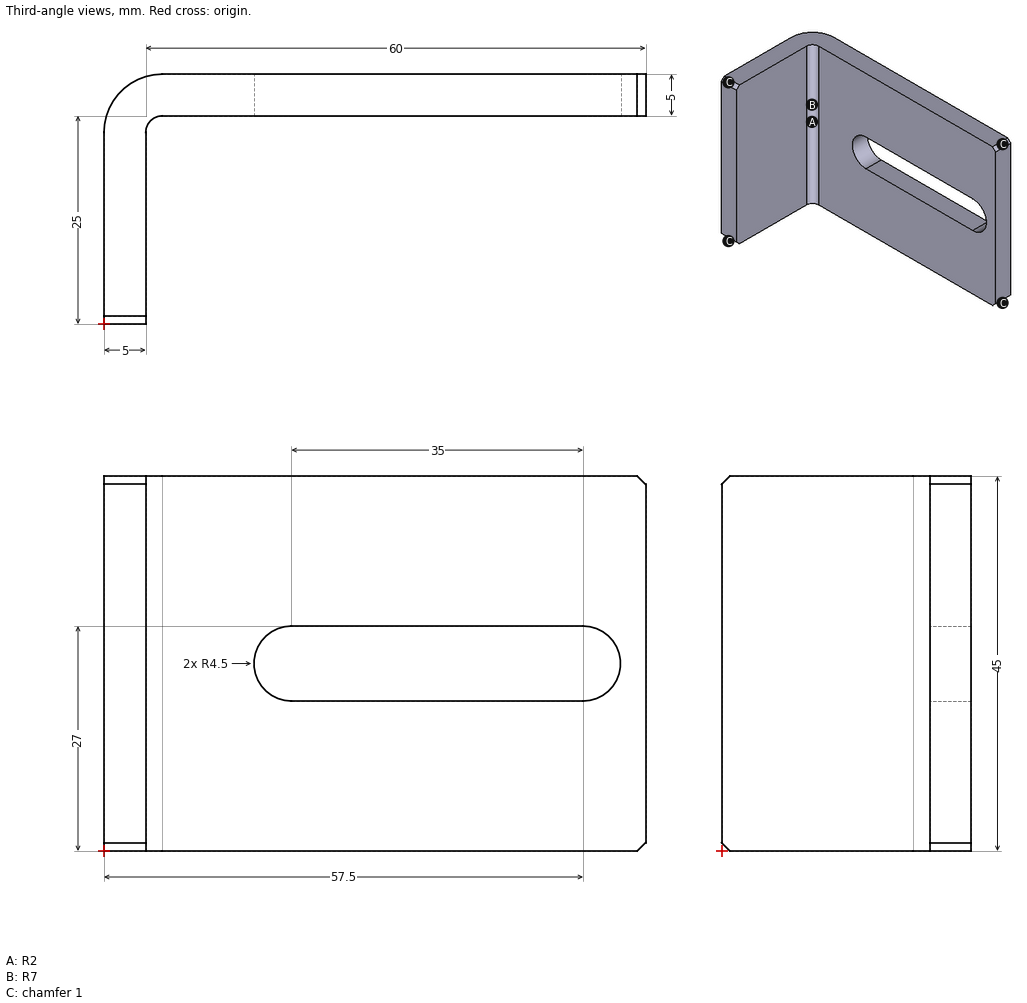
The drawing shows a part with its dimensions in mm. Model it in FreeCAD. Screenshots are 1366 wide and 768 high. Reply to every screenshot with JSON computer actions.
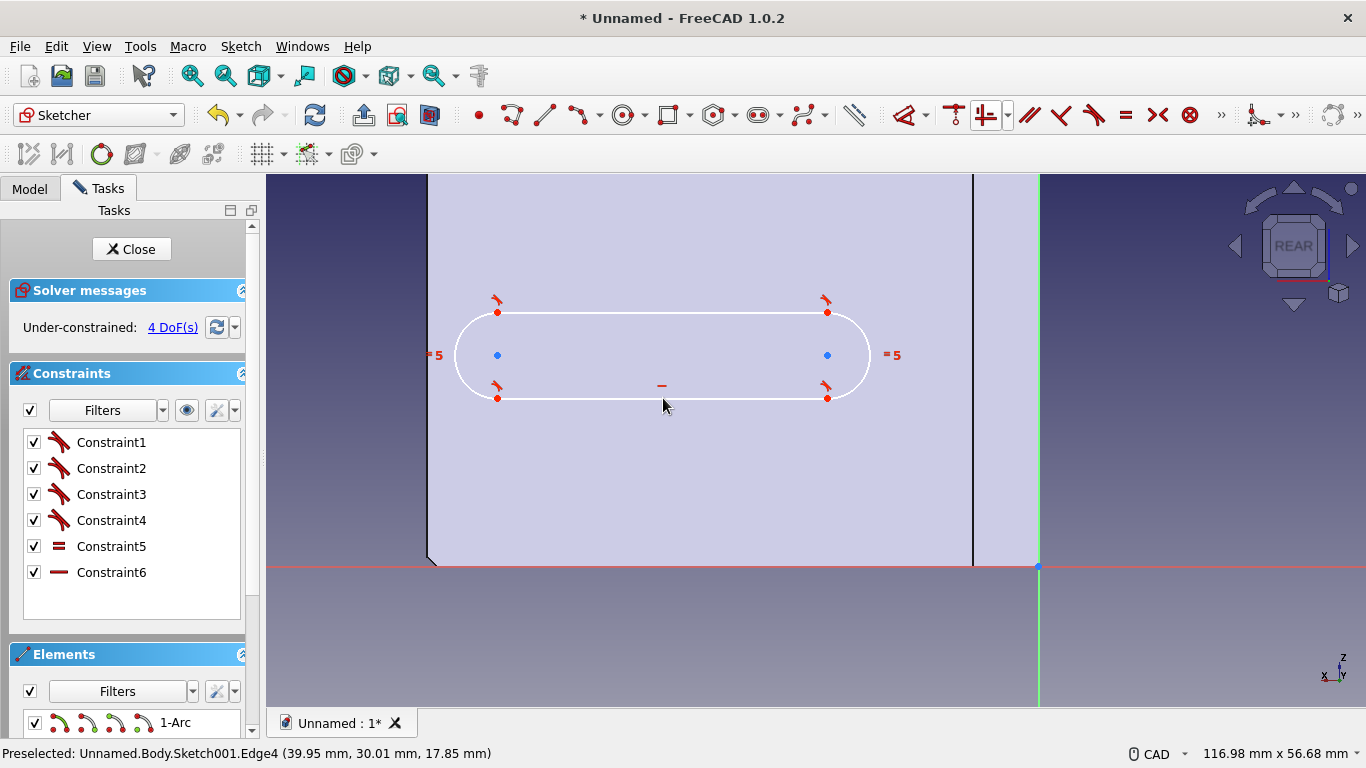
{"action": "key", "text": "d"}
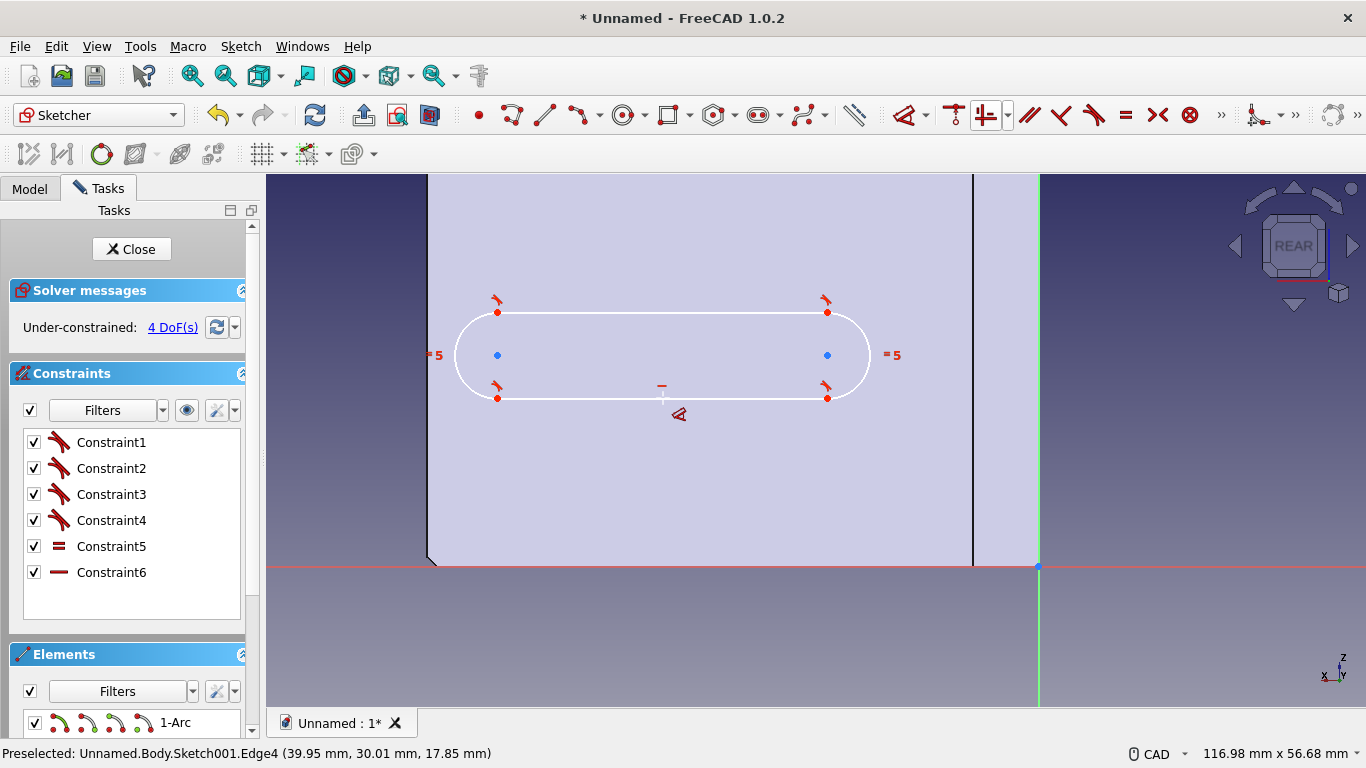
{"action": "left_click", "coordinate": [463, 331]}
{"action": "left_click", "coordinate": [437, 312]}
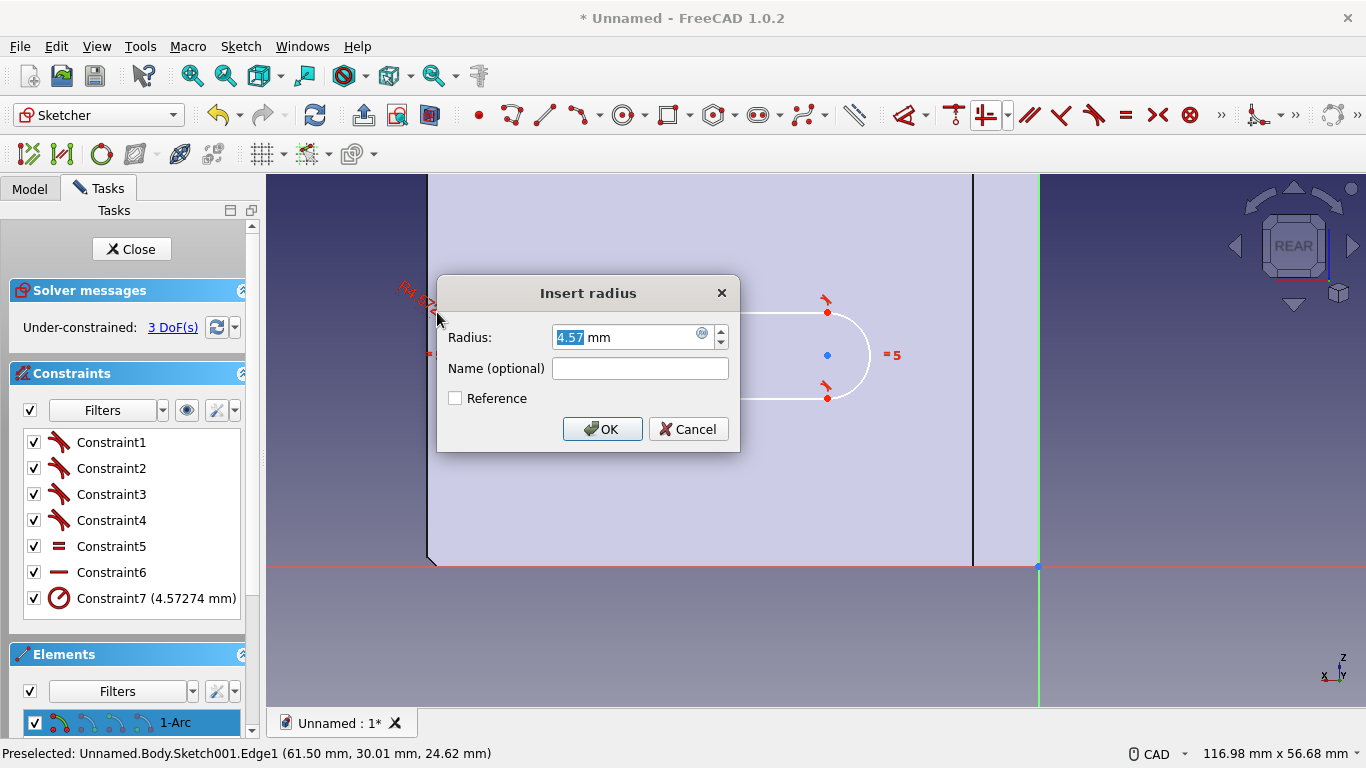
{"action": "type", "text": "4.5"}
{"action": "key", "text": "Return"}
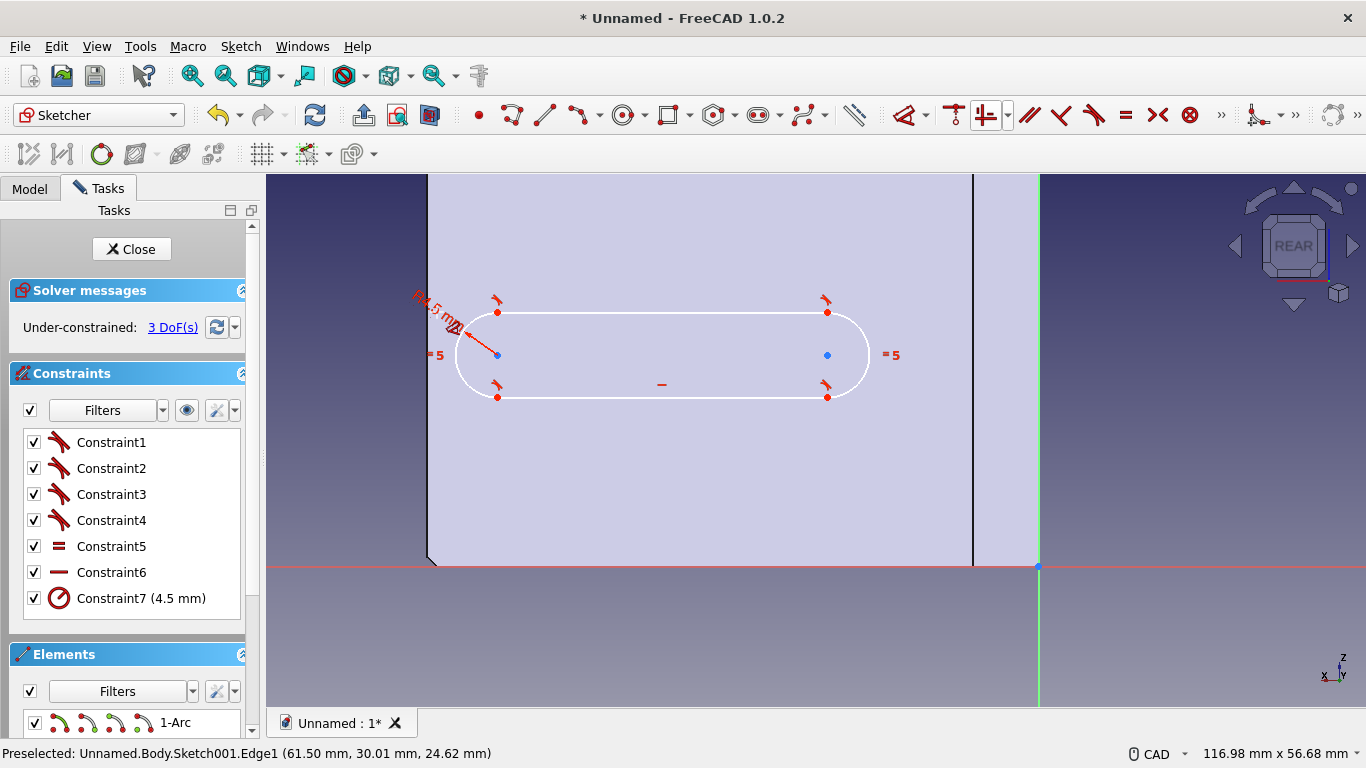
{"action": "left_click", "coordinate": [597, 313]}
{"action": "left_click", "coordinate": [662, 279]}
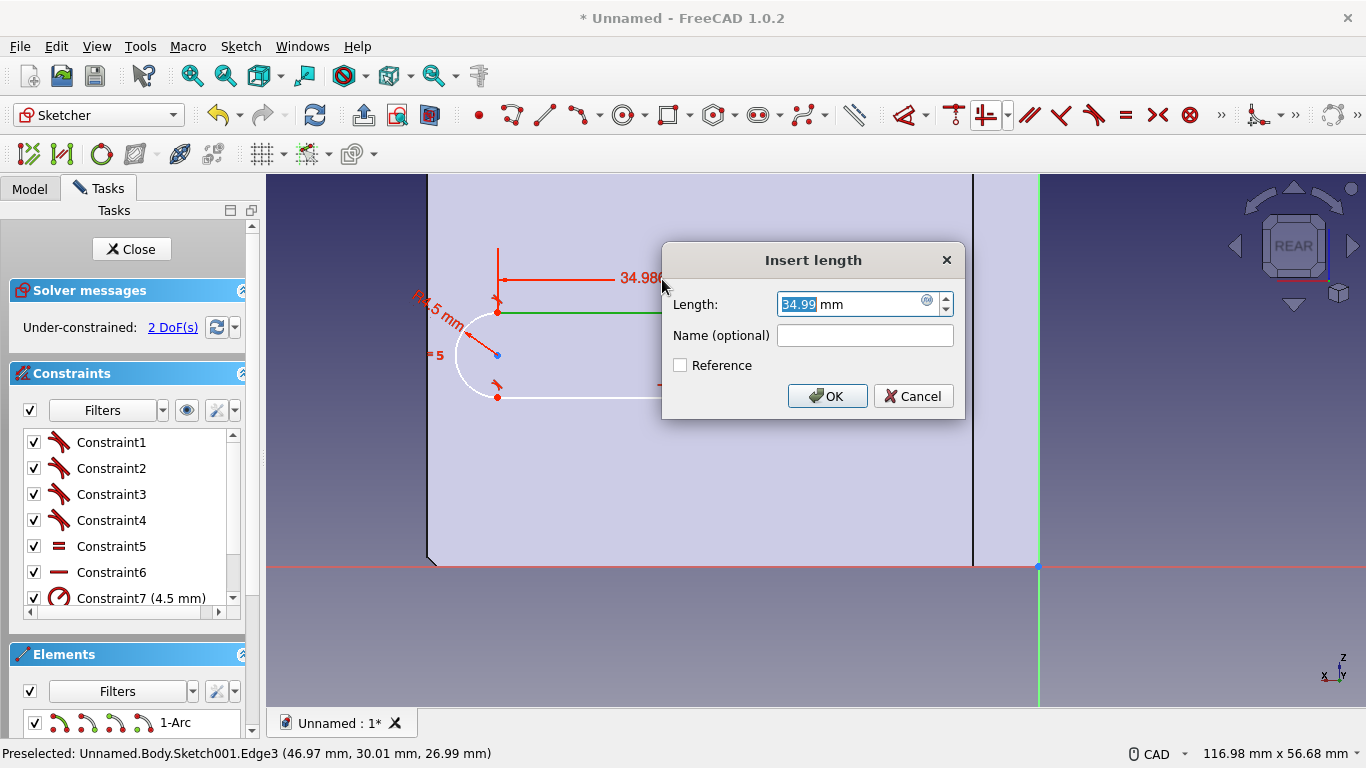
{"action": "type", "text": "35"}
{"action": "key", "text": "Return"}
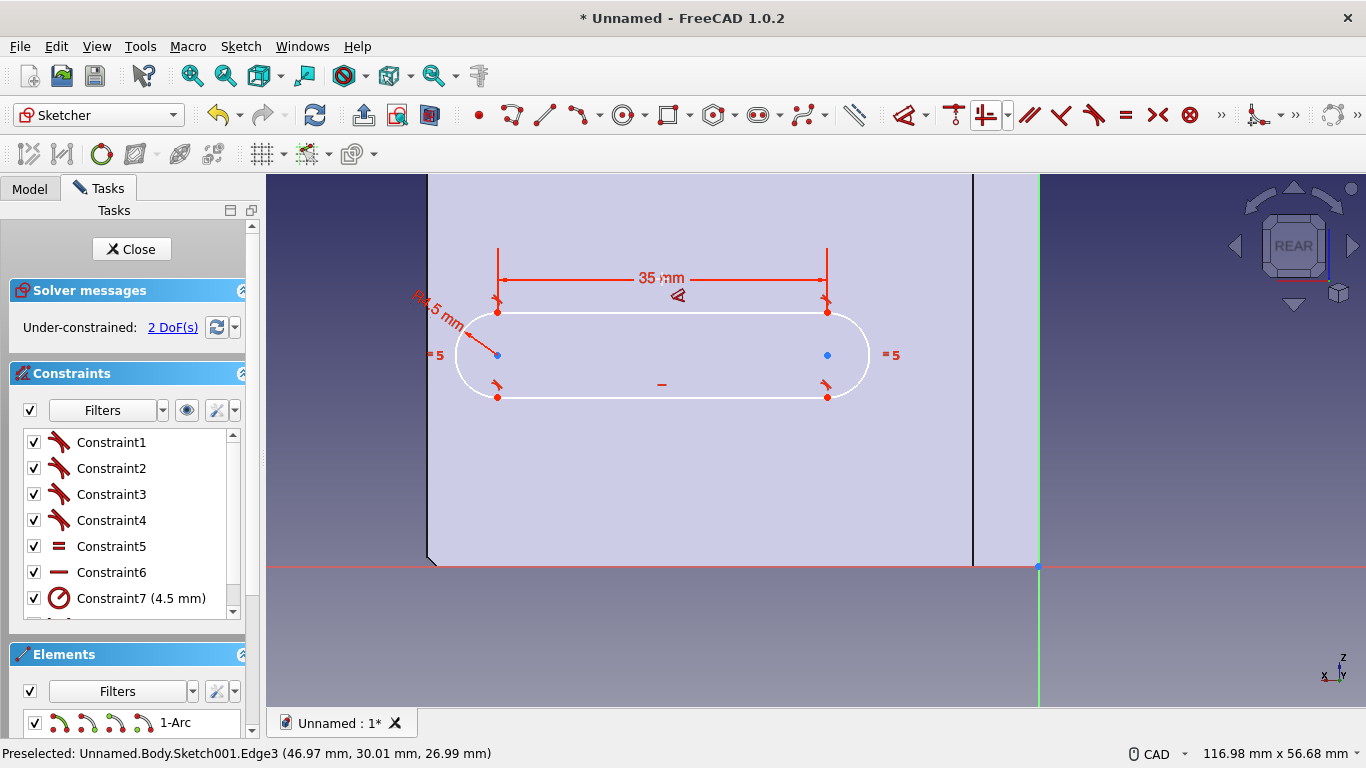
{"action": "left_click", "coordinate": [498, 313]}
{"action": "left_click", "coordinate": [1073, 440]}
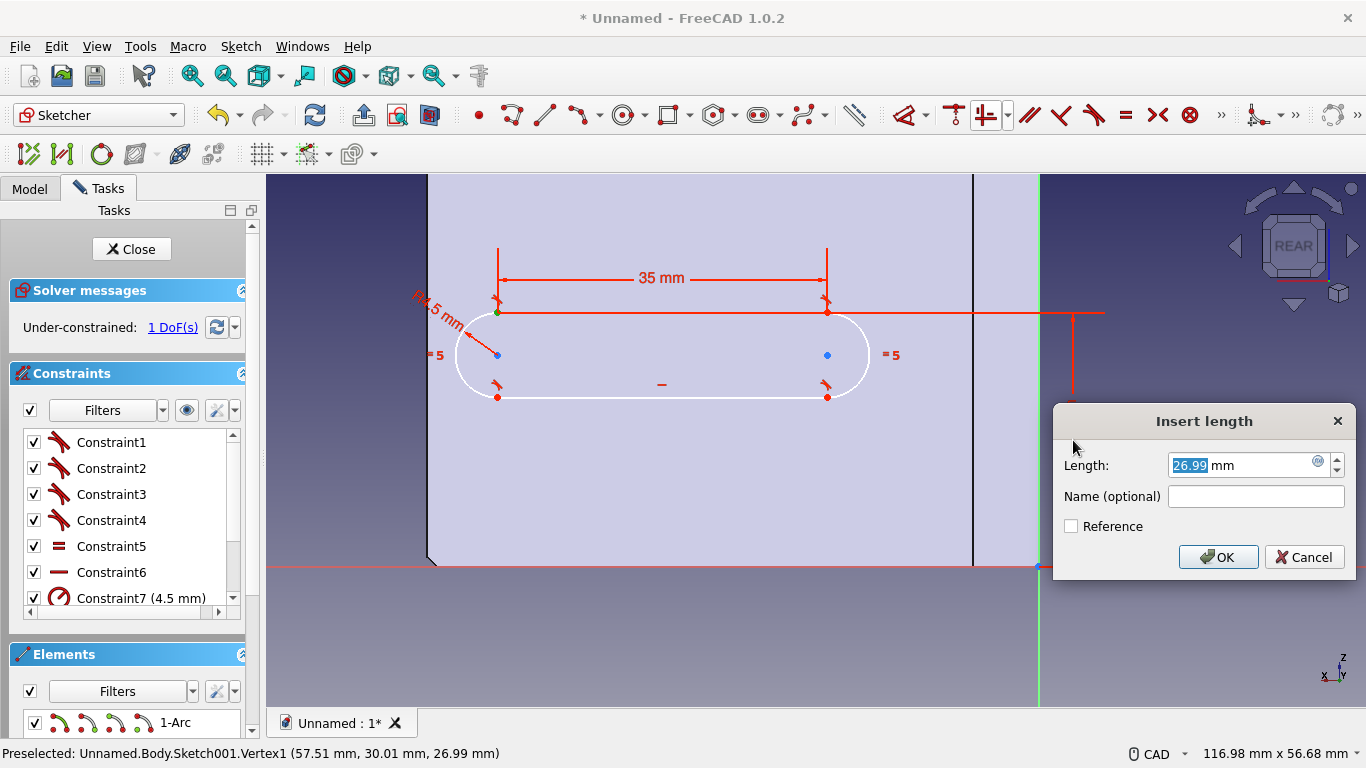
{"action": "type", "text": "27"}
{"action": "key", "text": "Return"}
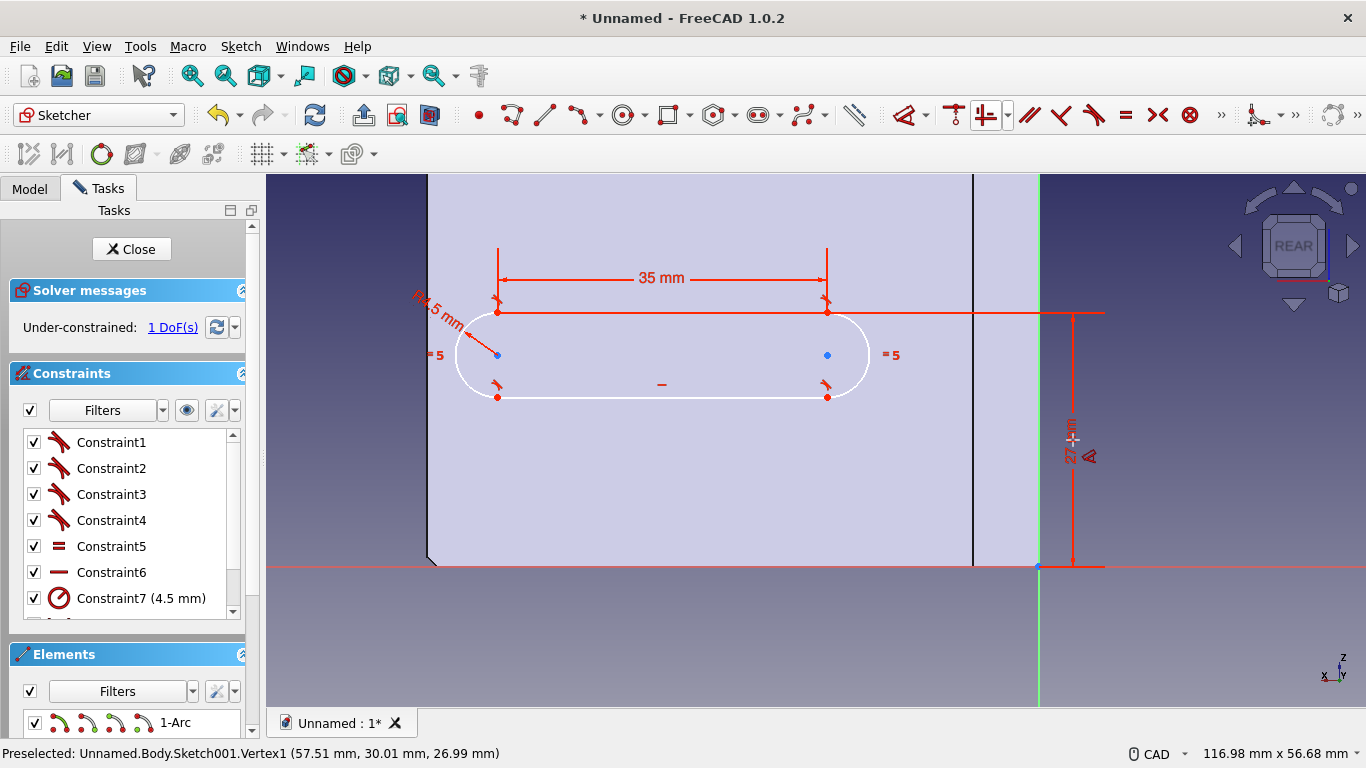
{"action": "left_click", "coordinate": [498, 313]}
{"action": "left_click", "coordinate": [768, 601]}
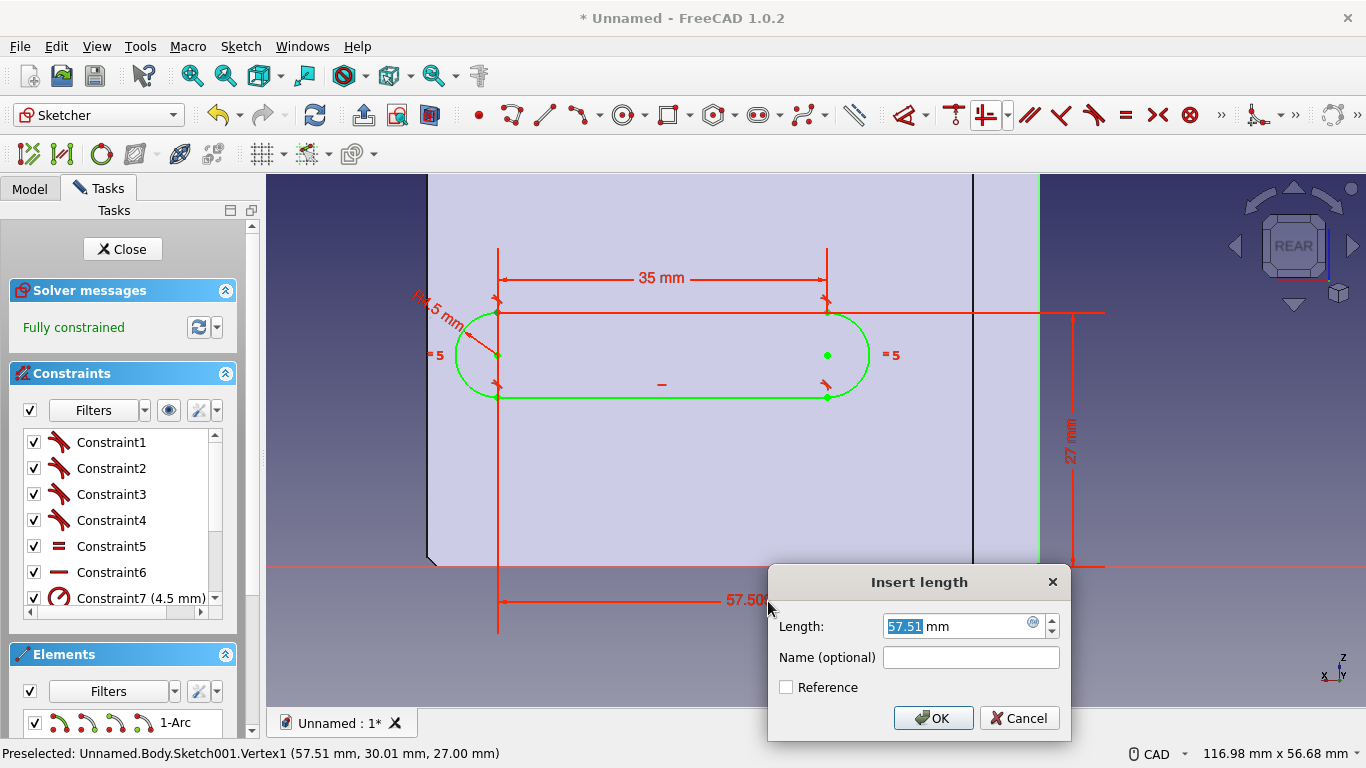
{"action": "type", "text": "57.5"}
{"action": "key", "text": "Return"}
{"action": "key", "text": "Escape"}